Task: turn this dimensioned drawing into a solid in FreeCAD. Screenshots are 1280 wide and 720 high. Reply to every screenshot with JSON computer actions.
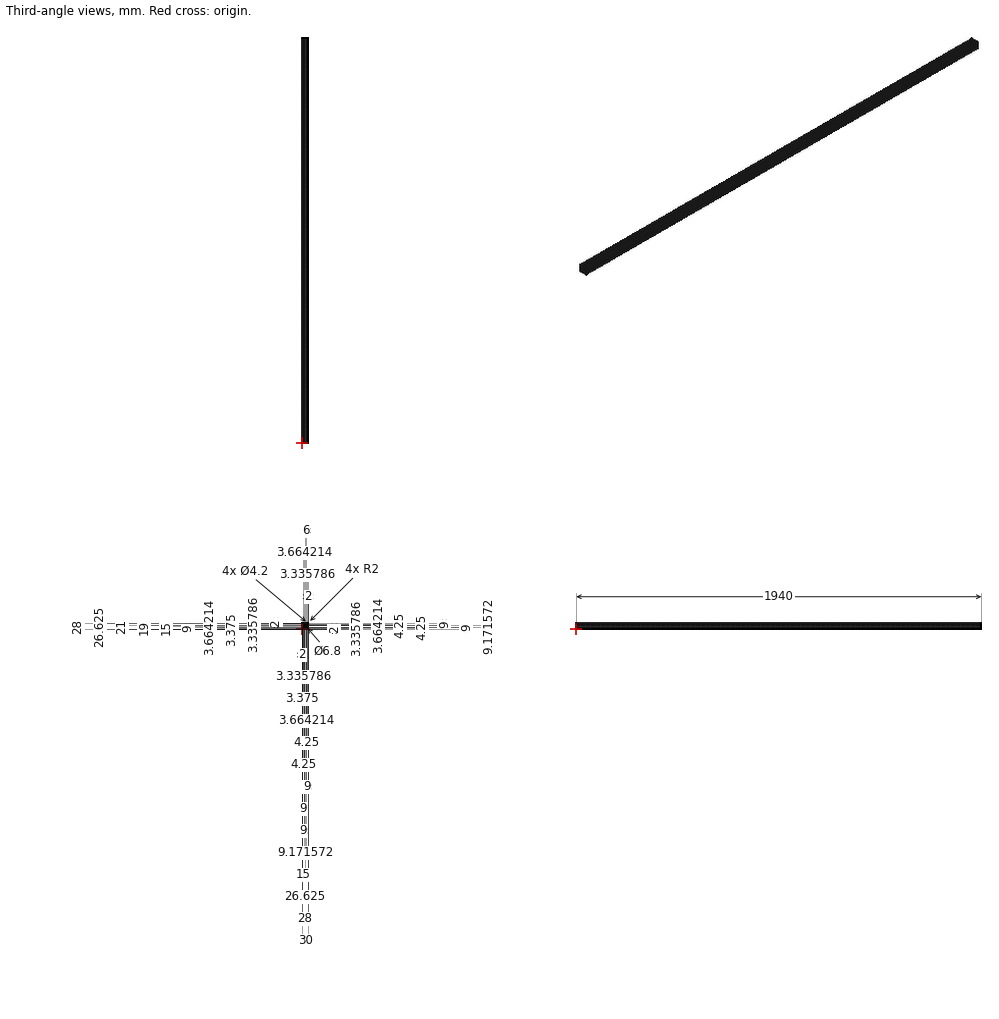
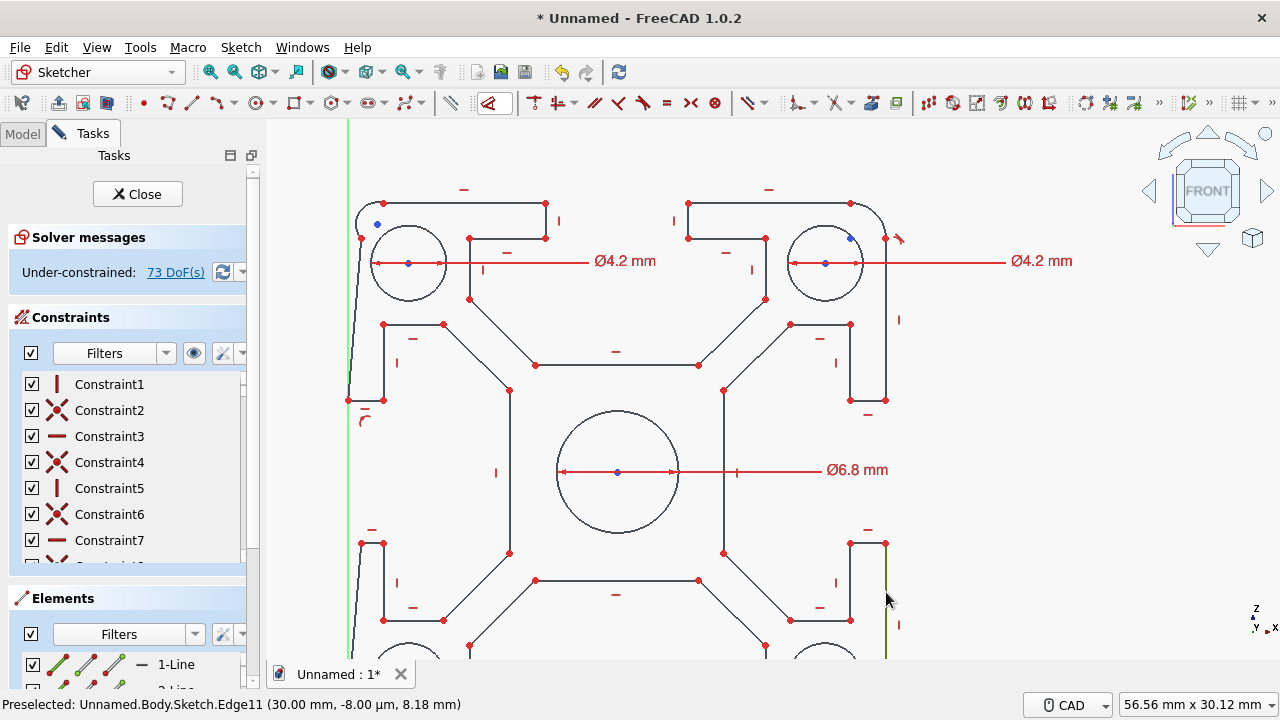
{"action": "scroll", "coordinate": [882, 223], "scroll_direction": "down", "scroll_amount": 2}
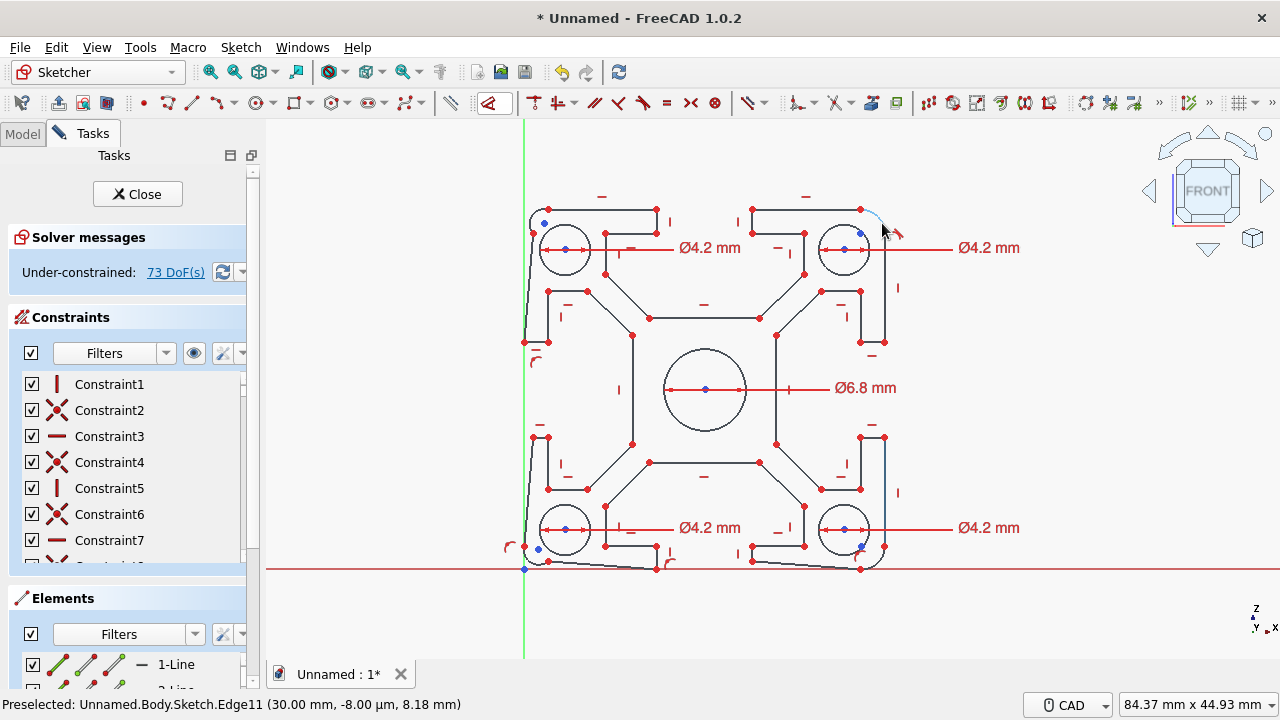
{"action": "scroll", "coordinate": [872, 567], "scroll_direction": "up", "scroll_amount": 2}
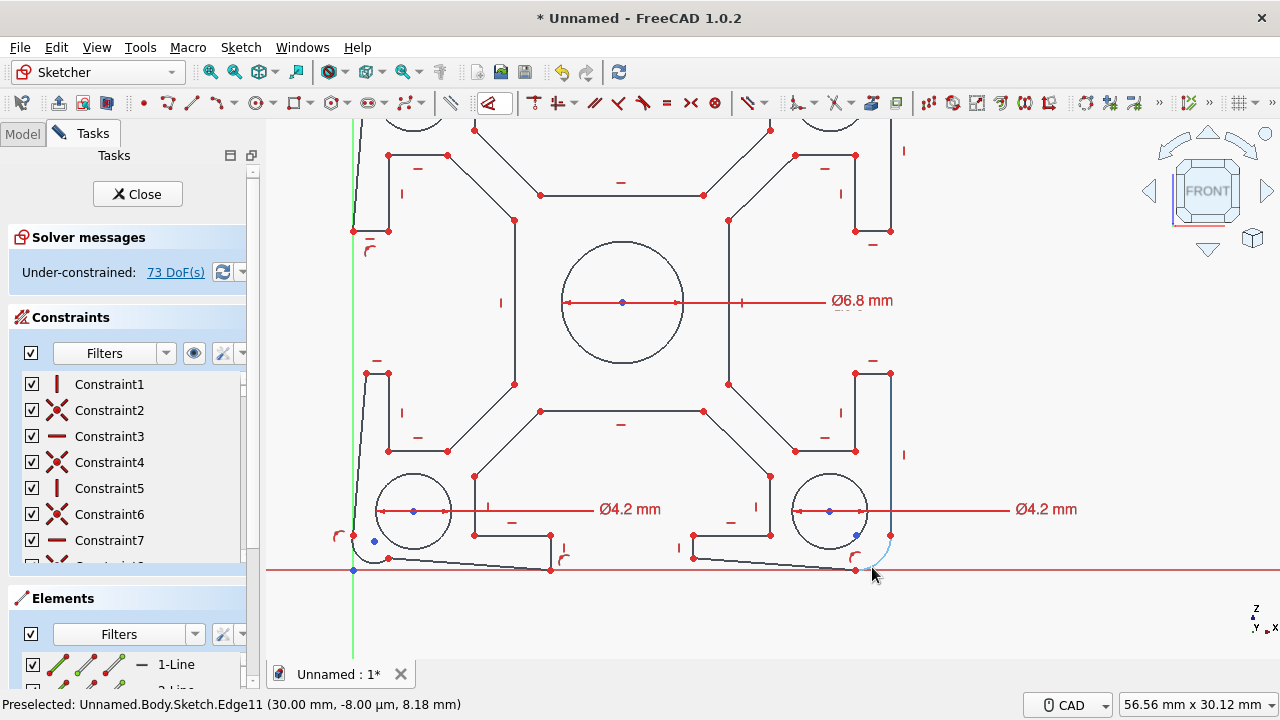
{"action": "left_click", "coordinate": [871, 567]}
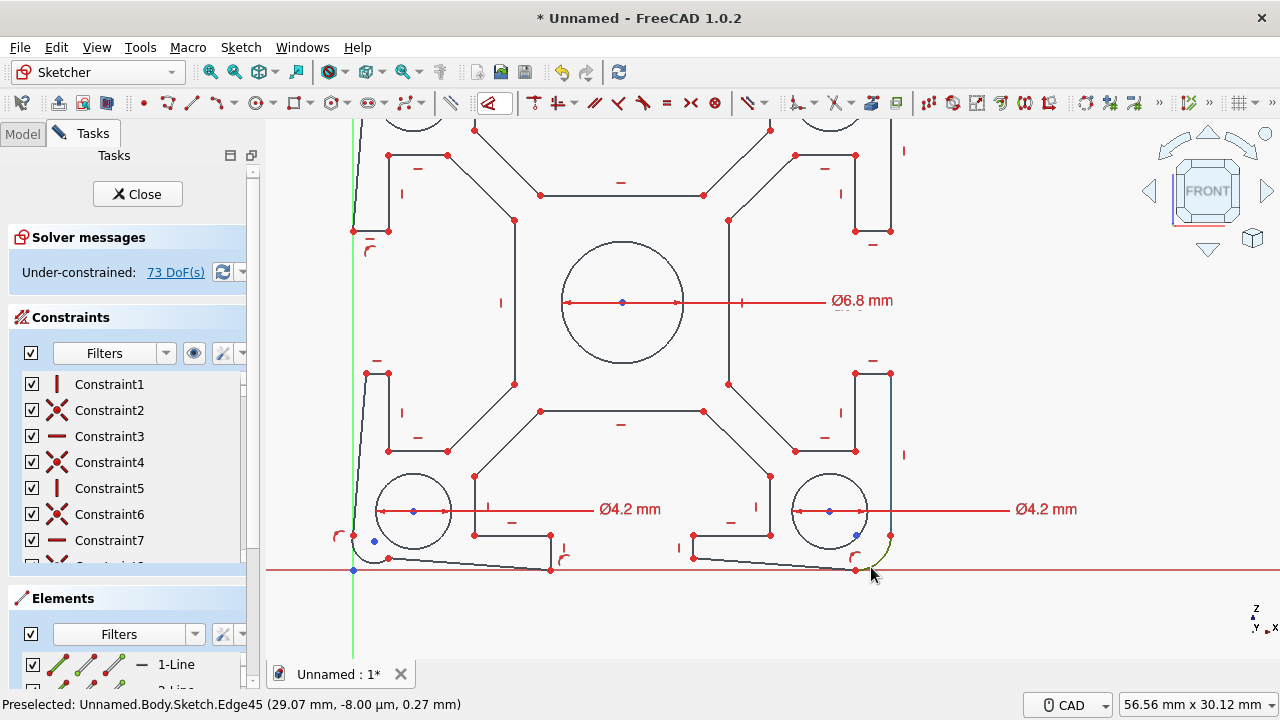
{"action": "key", "text": "t"}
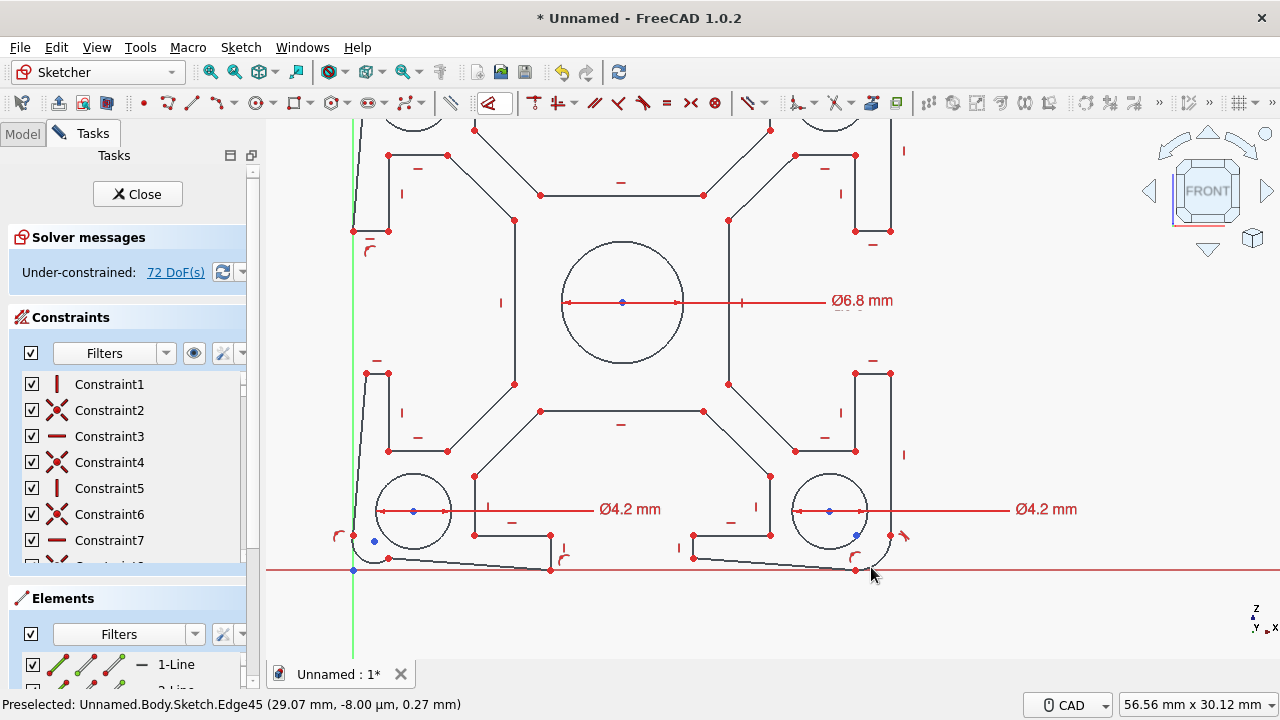
{"action": "left_click", "coordinate": [807, 567]}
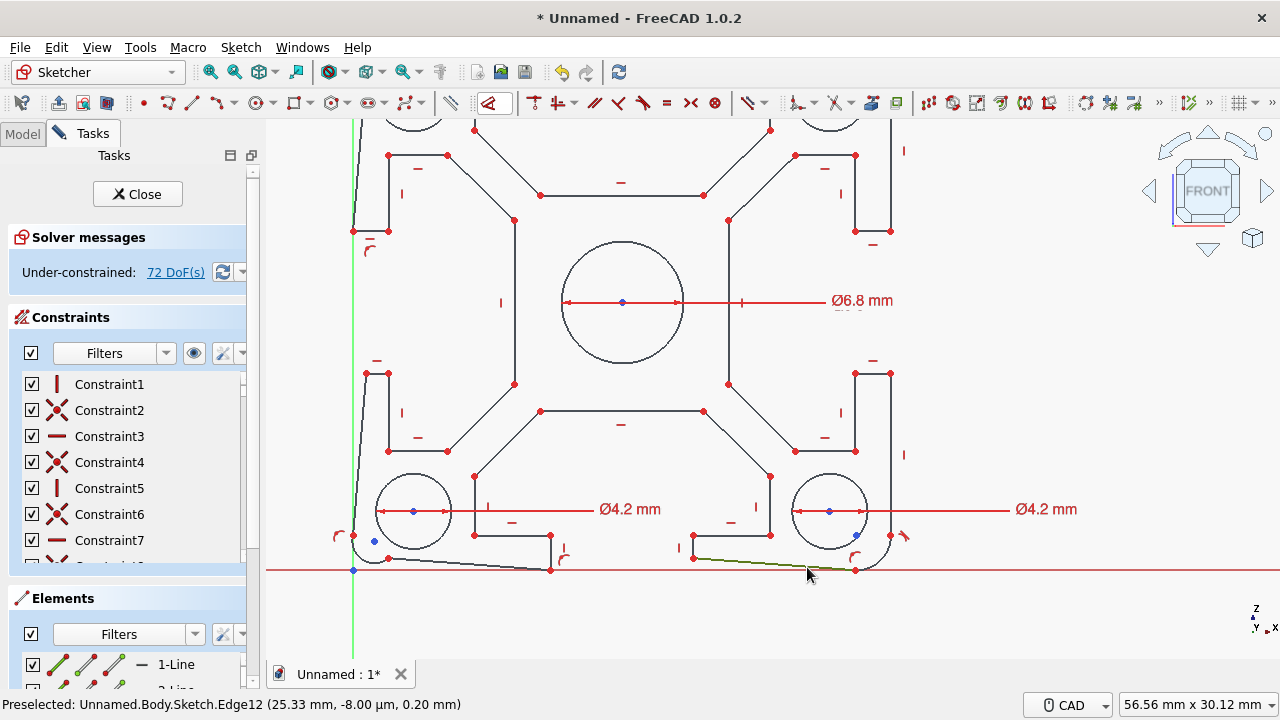
{"action": "left_click", "coordinate": [871, 567]}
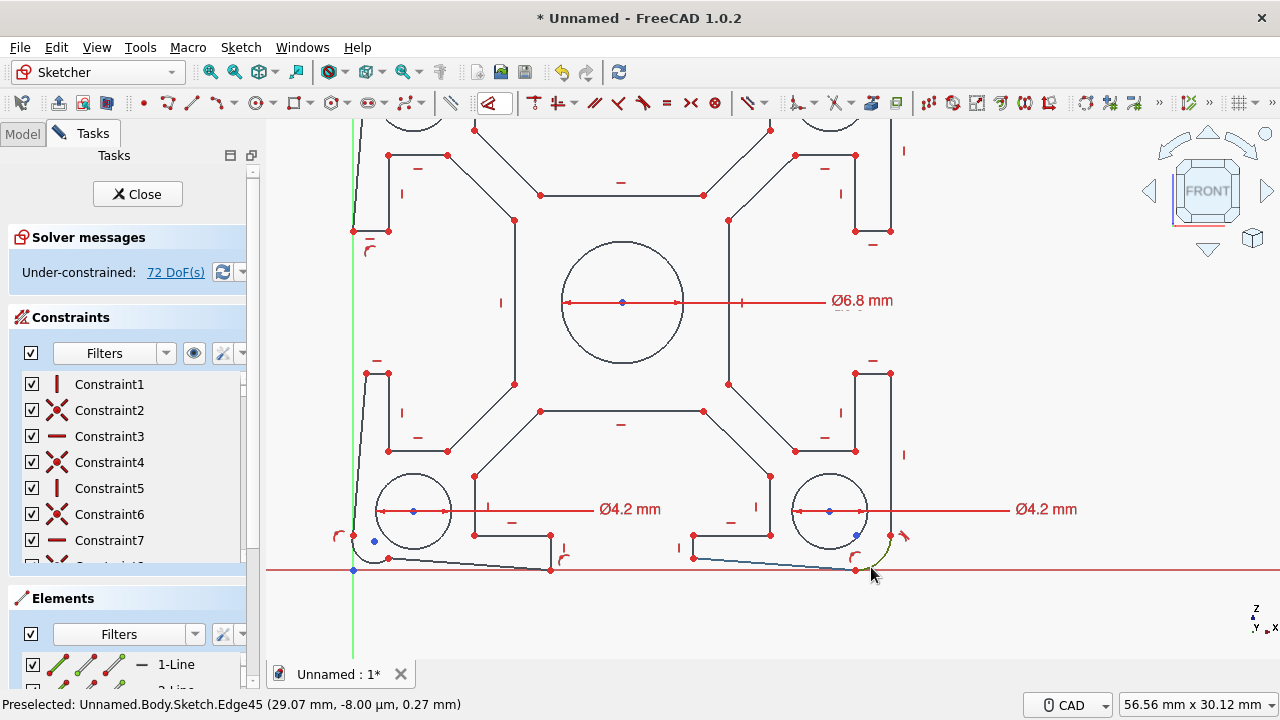
{"action": "key", "text": "t"}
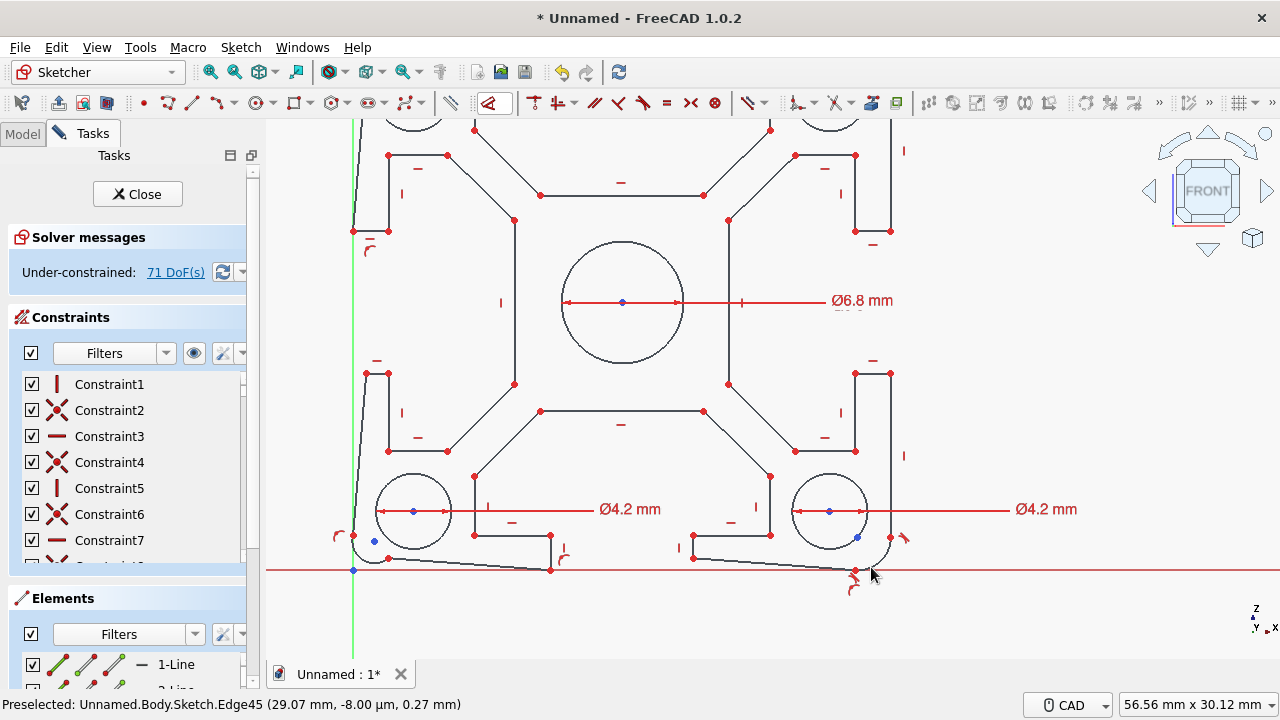
{"action": "left_click", "coordinate": [502, 567]}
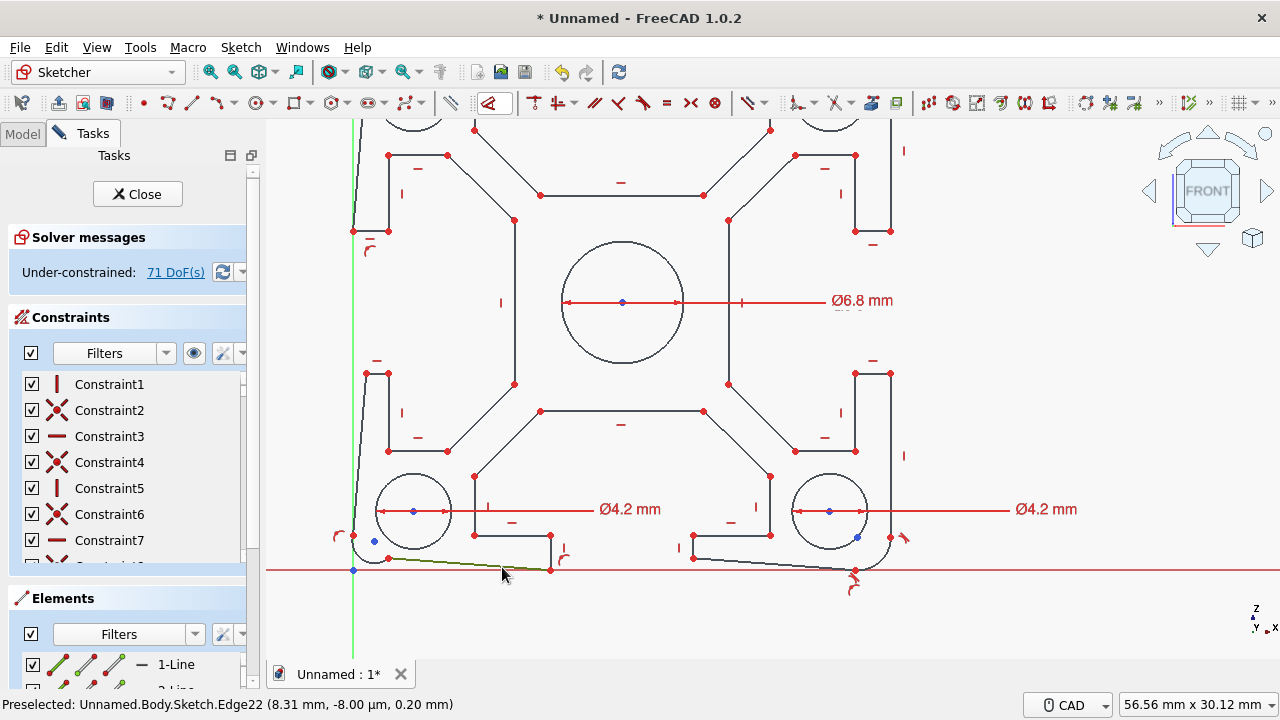
{"action": "left_click", "coordinate": [355, 552]}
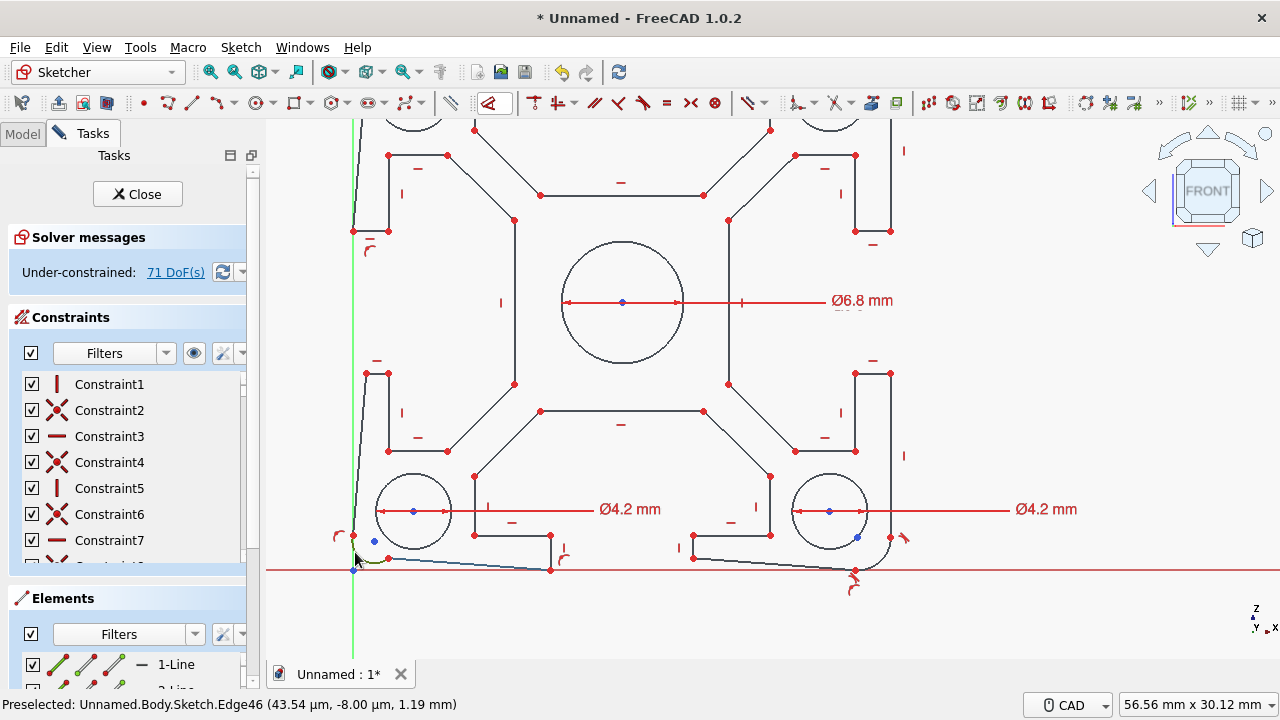
{"action": "key", "text": "t"}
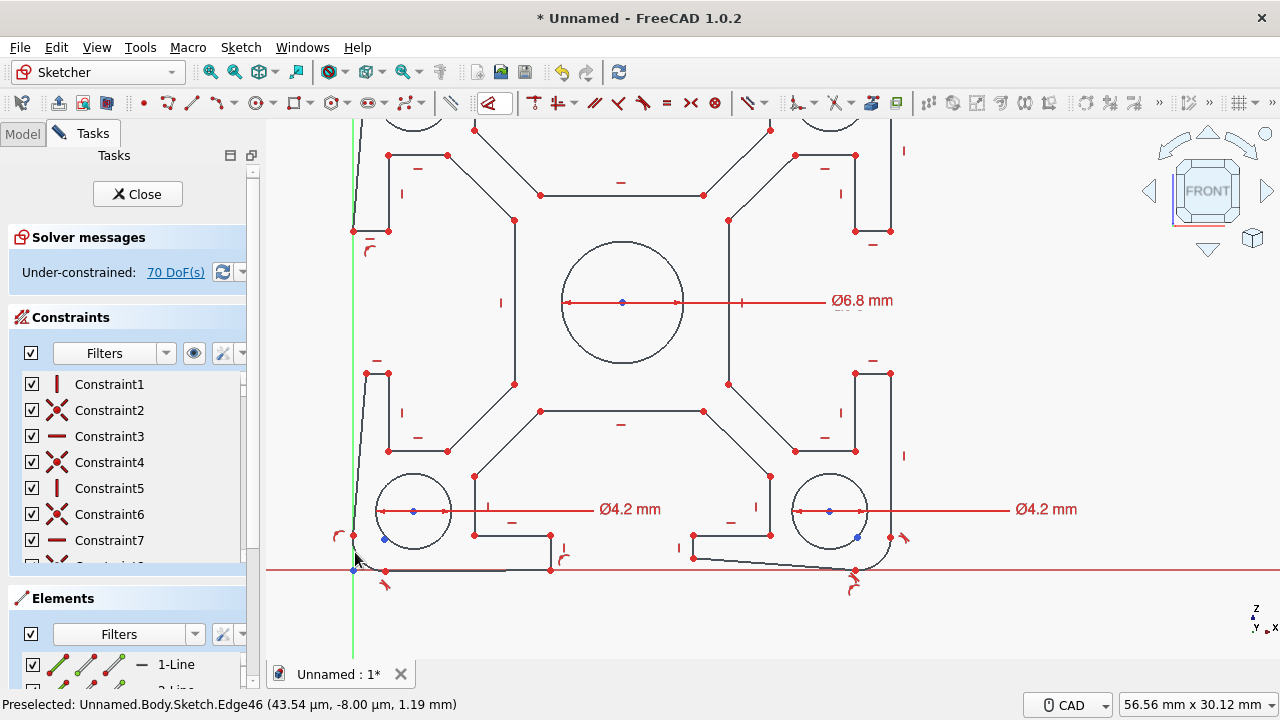
{"action": "left_click", "coordinate": [357, 487]}